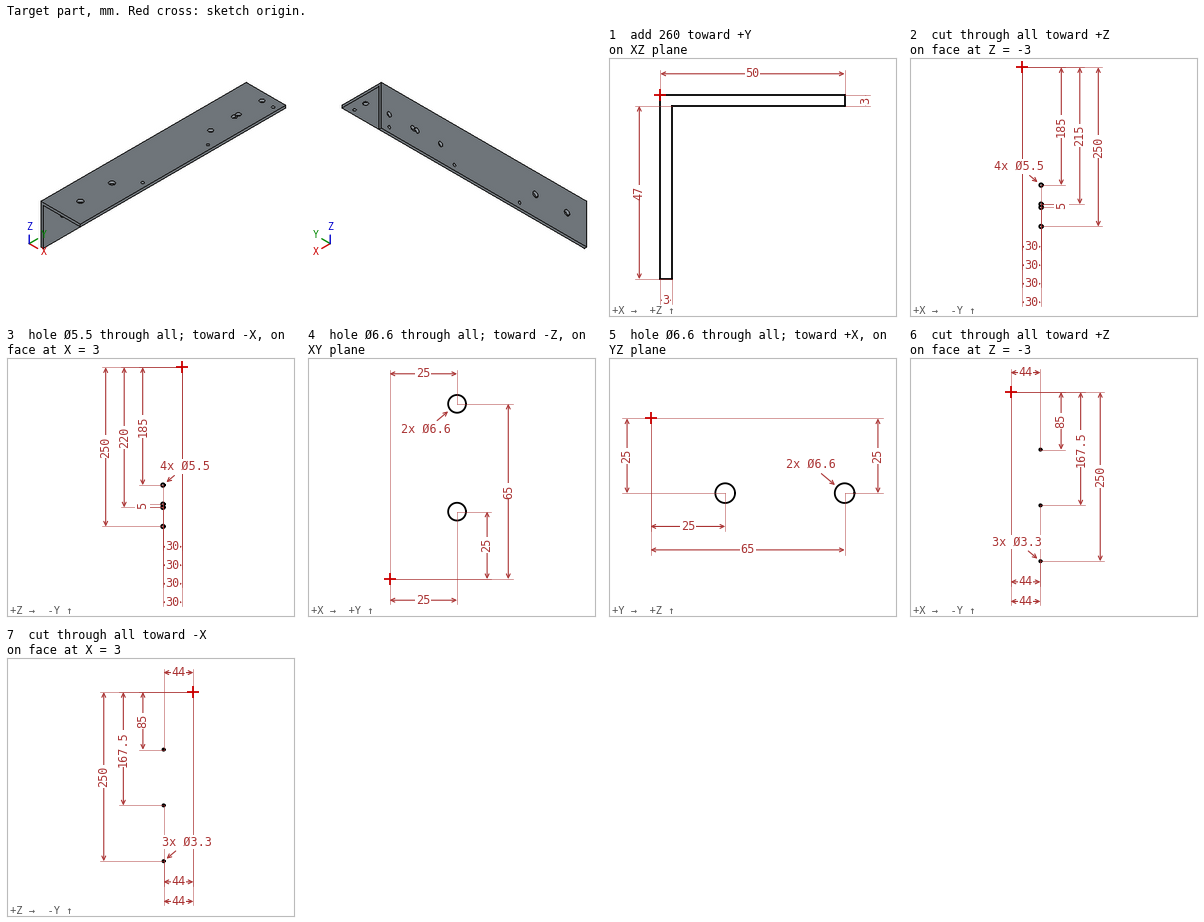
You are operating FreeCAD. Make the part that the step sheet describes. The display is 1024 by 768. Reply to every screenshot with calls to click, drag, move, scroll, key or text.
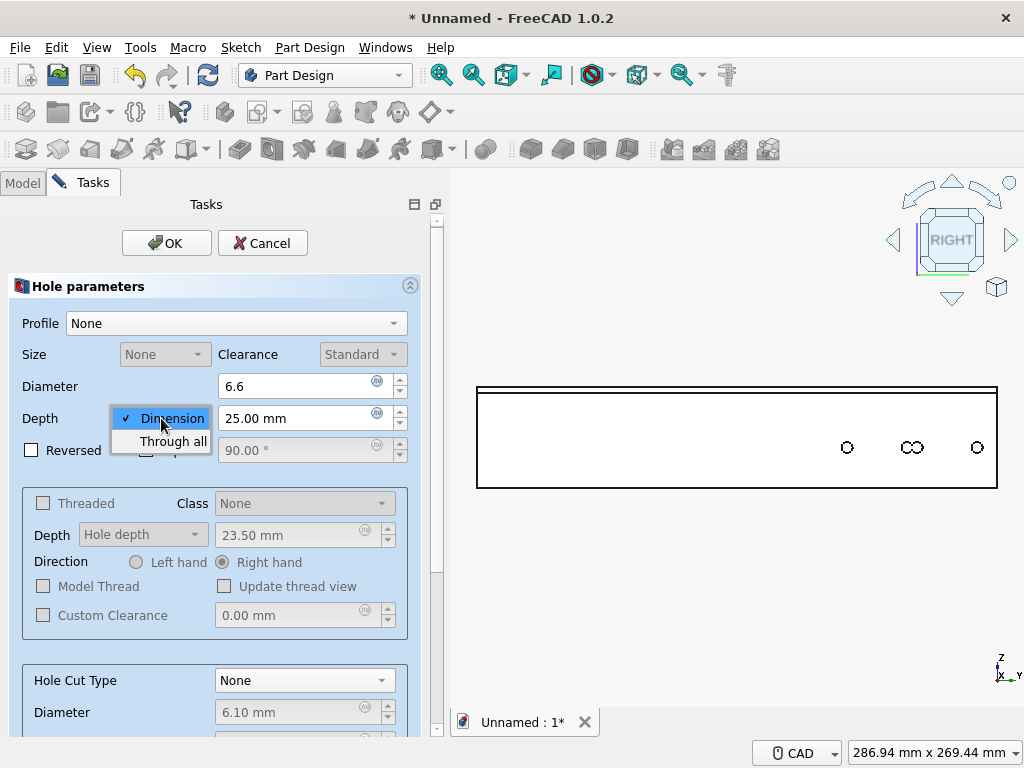
click(160, 442)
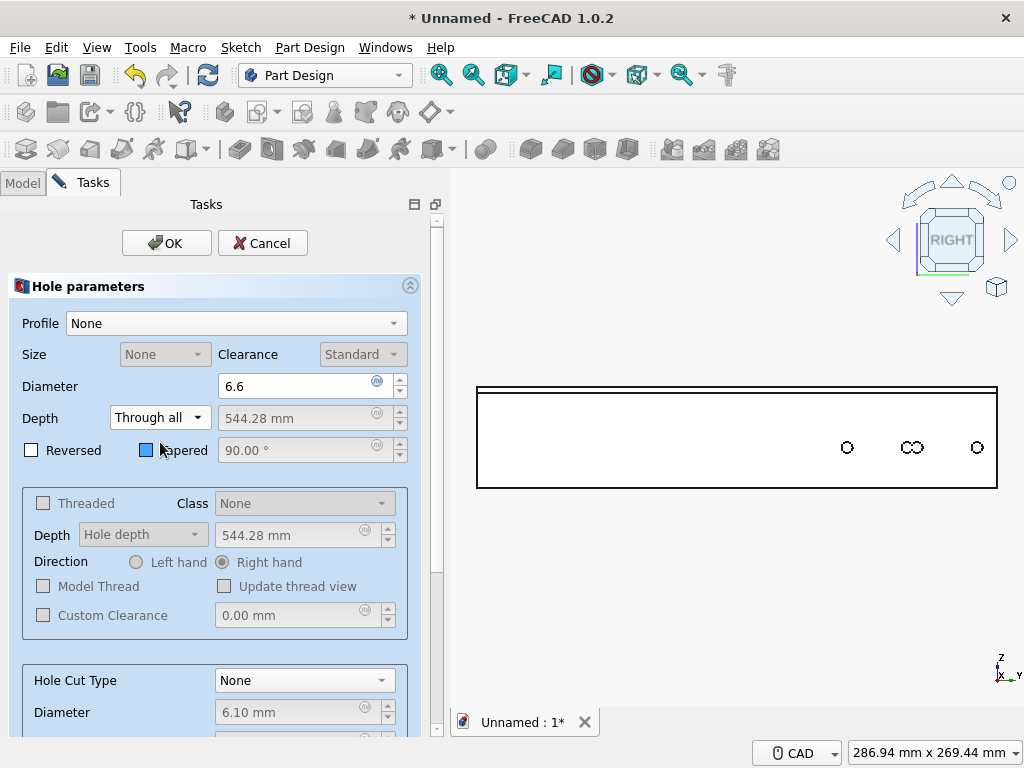
click(167, 243)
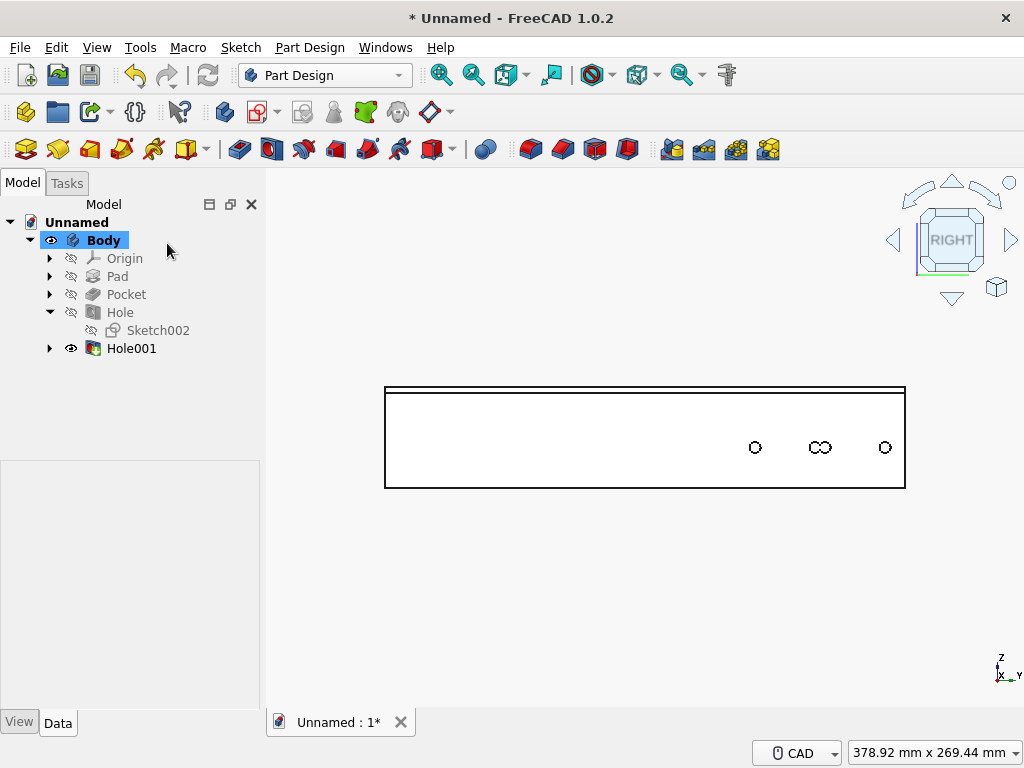
click(258, 112)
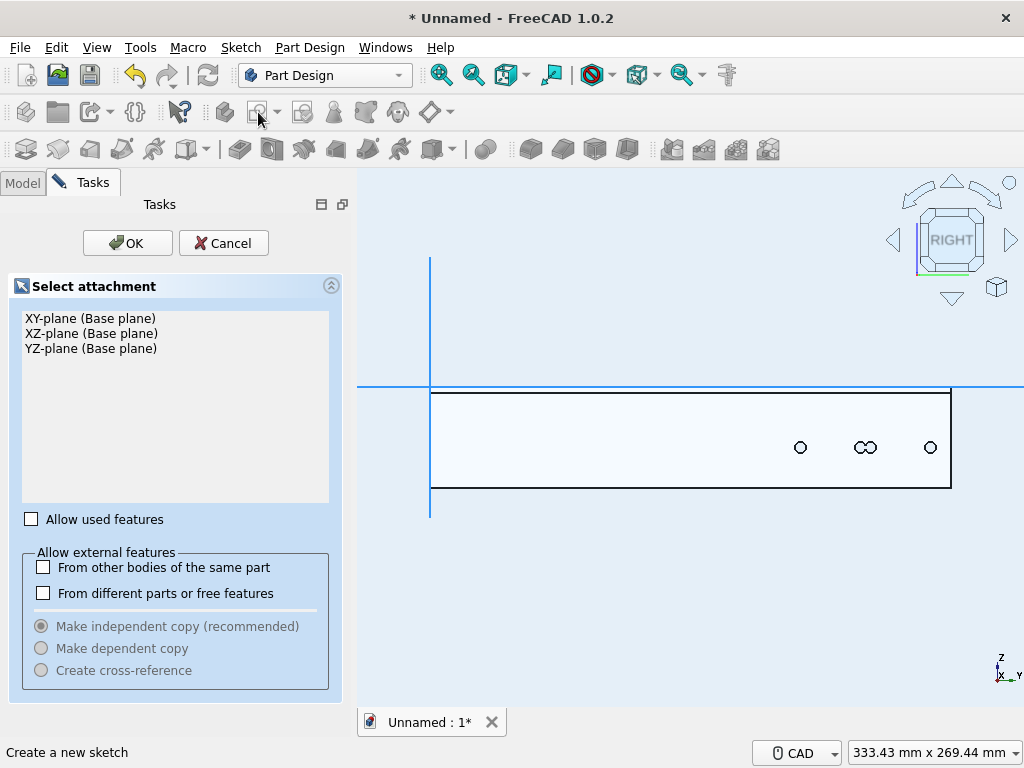
click(82, 348)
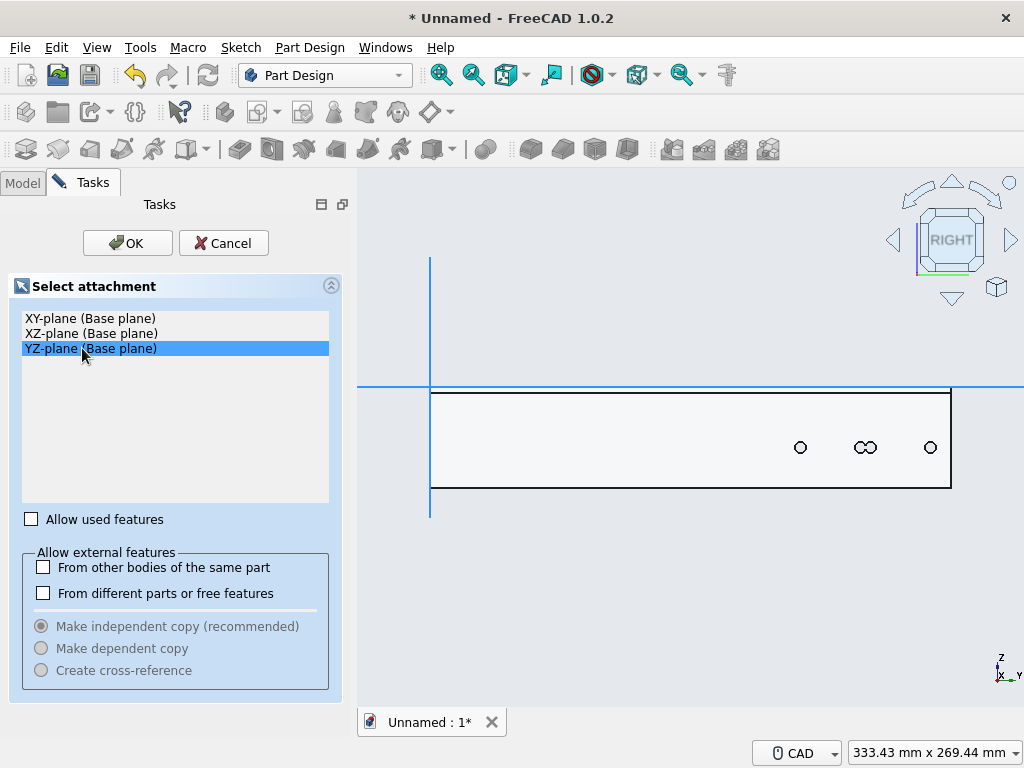
click(128, 243)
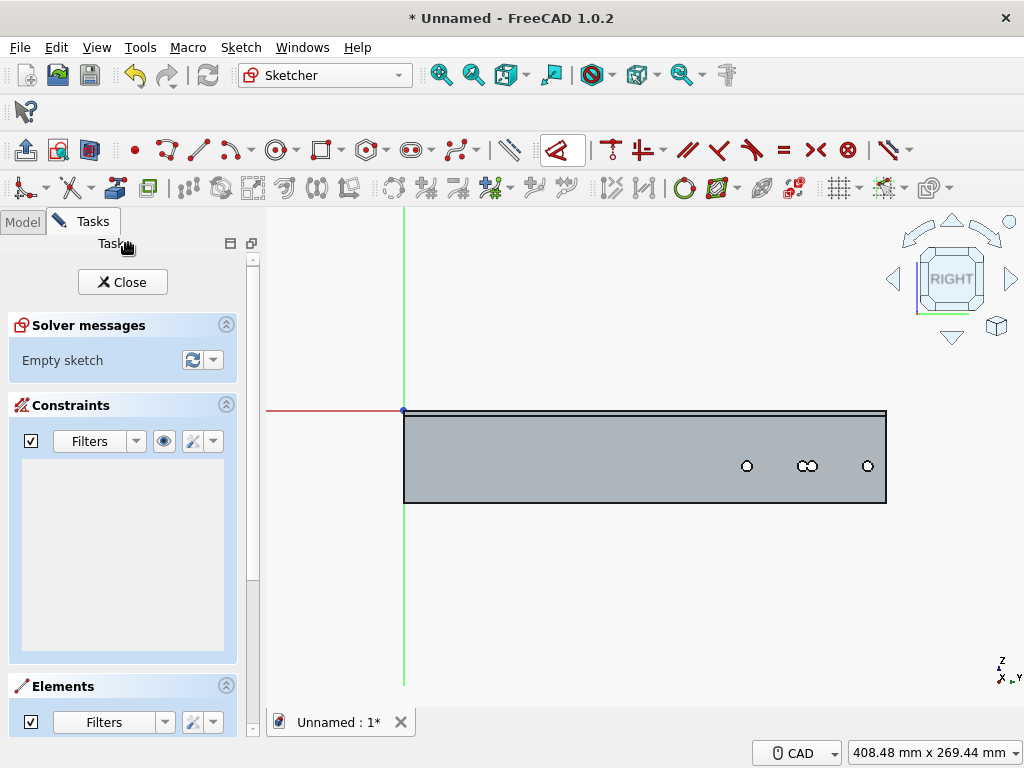
key(q)
key(s)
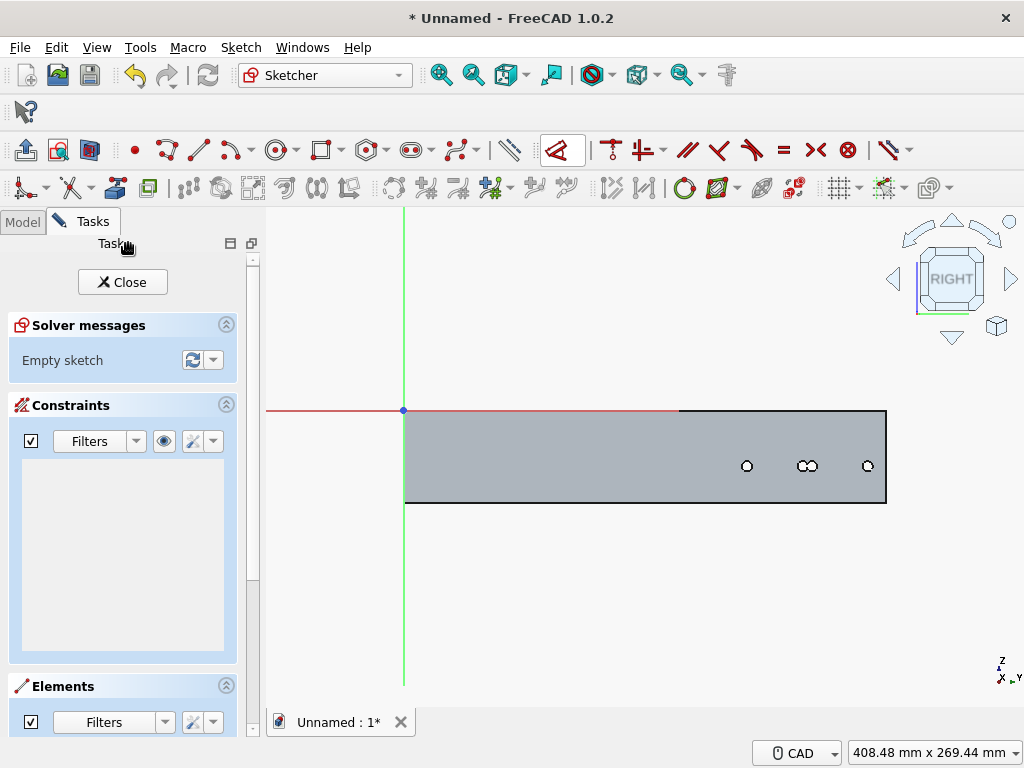
scroll(420, 428, up, 6)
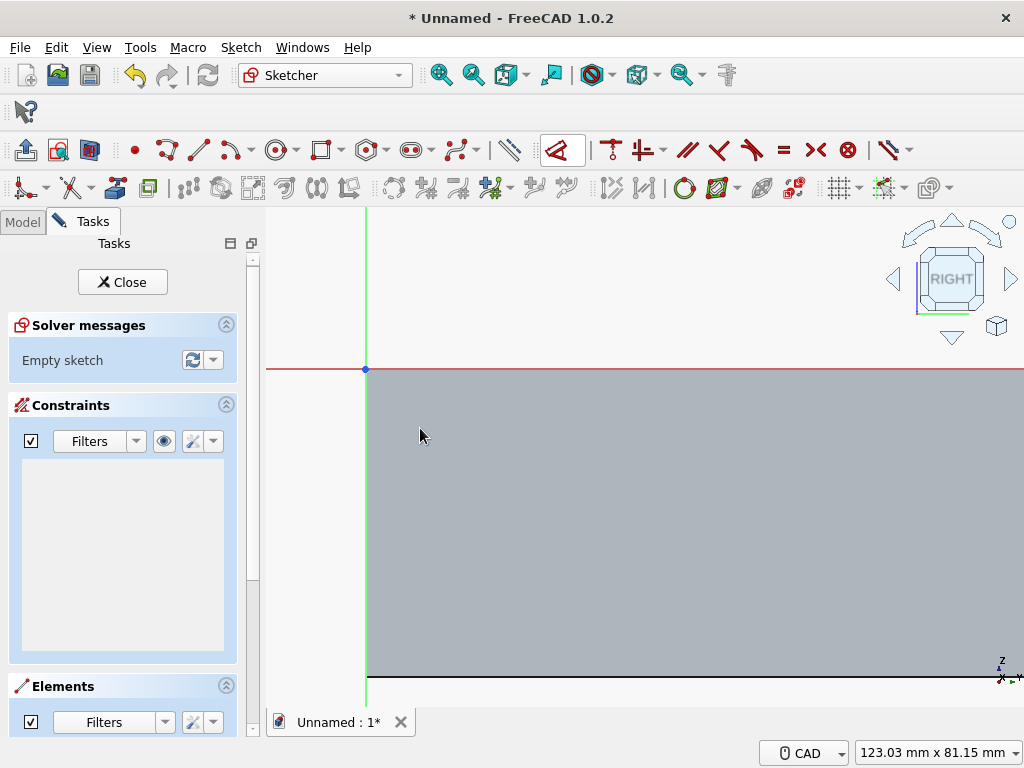
key(g)
key(c)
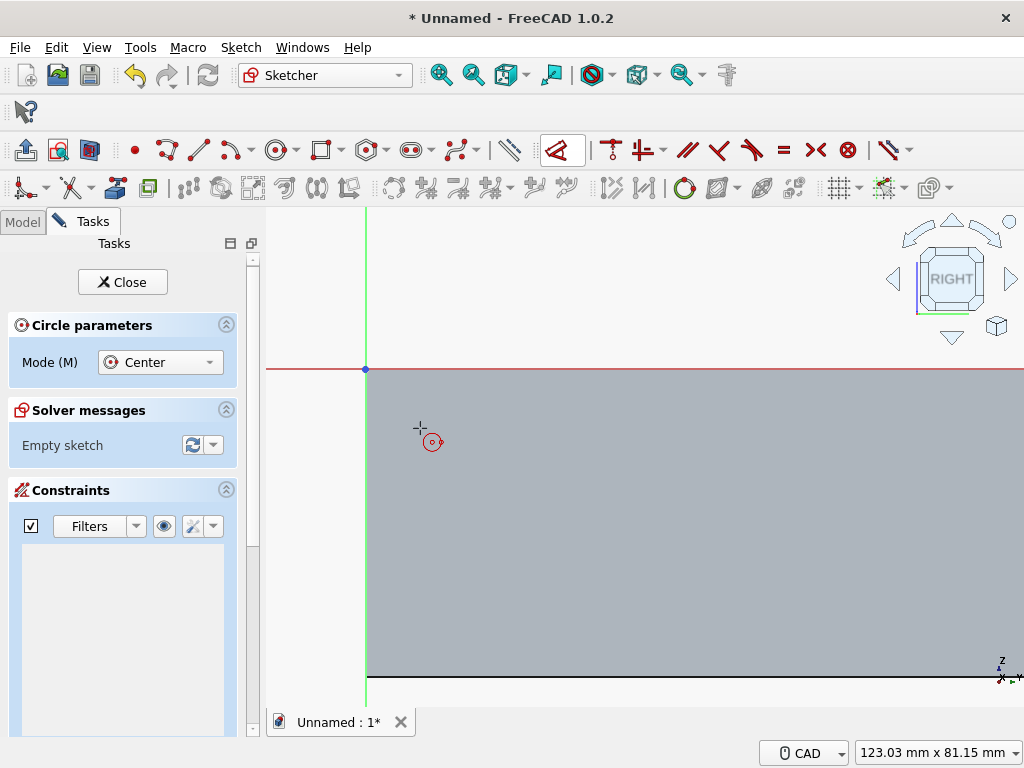
click(766, 523)
click(780, 509)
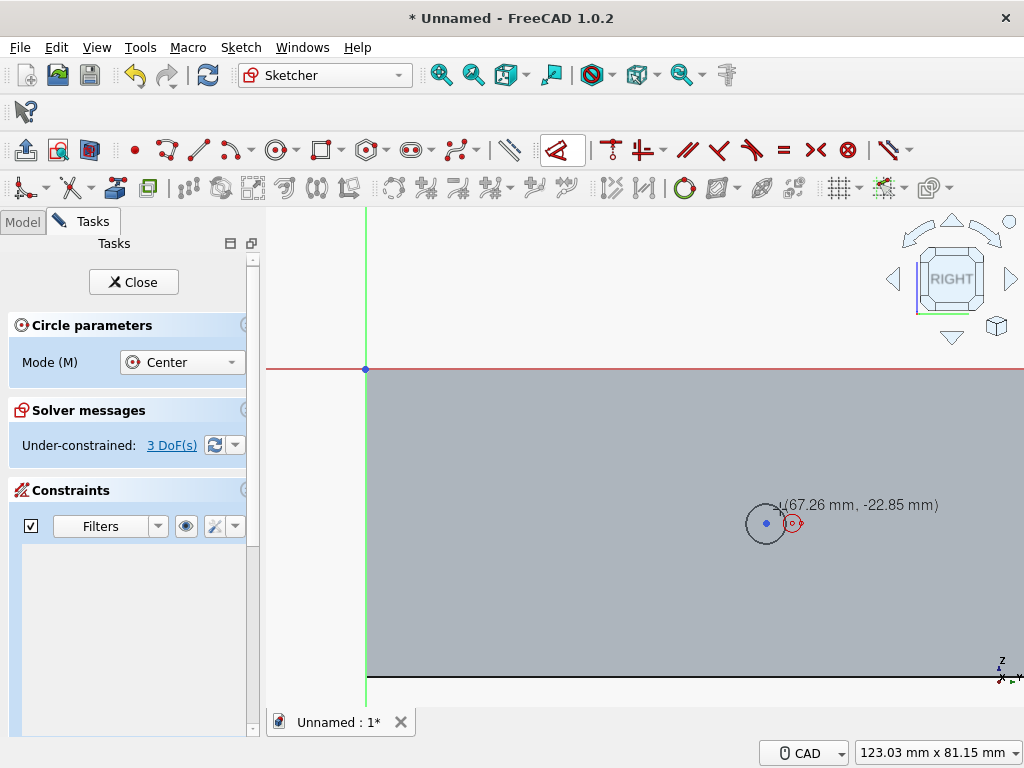
click(520, 523)
click(534, 509)
key(Escape)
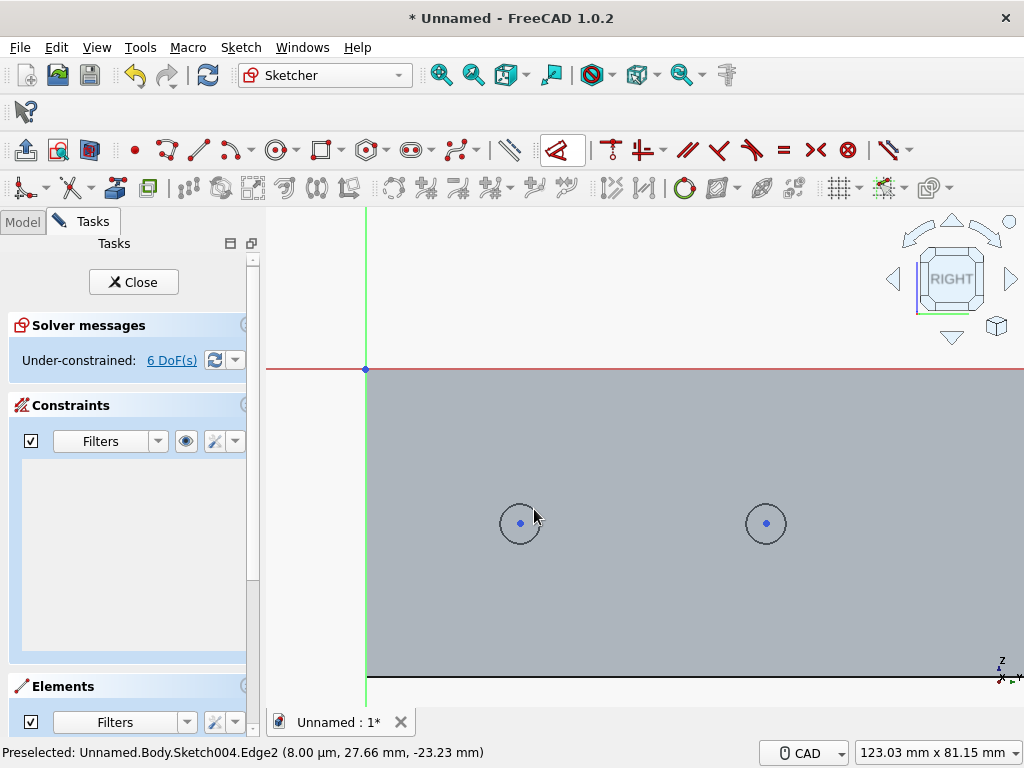
click(780, 510)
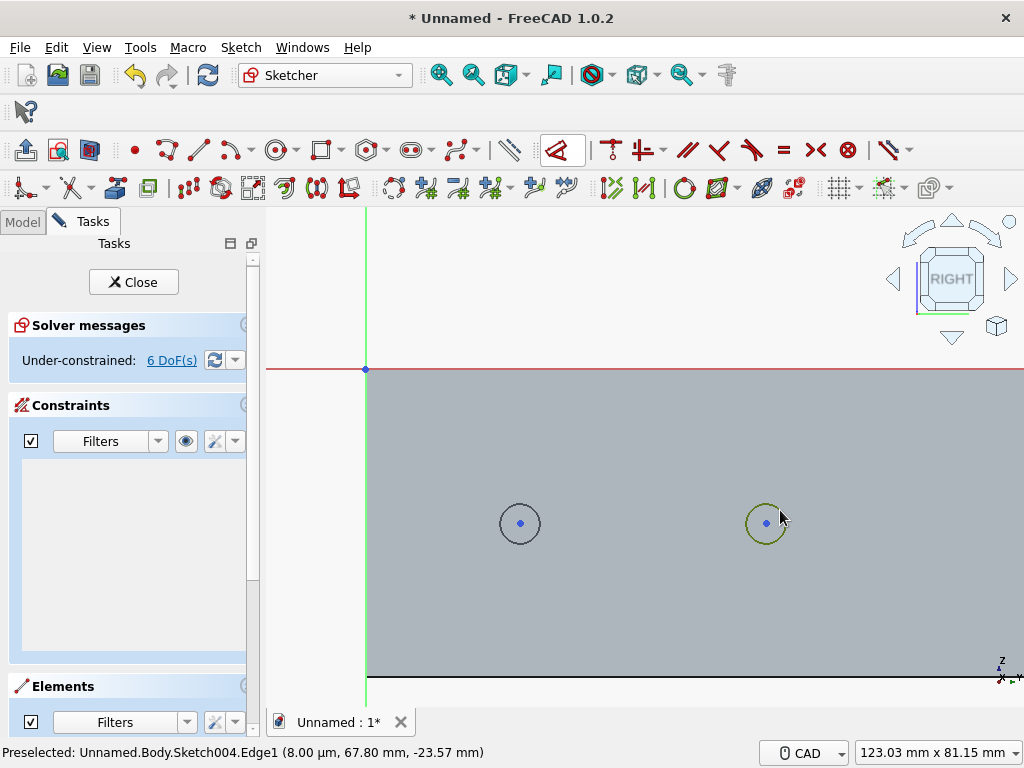
click(534, 510)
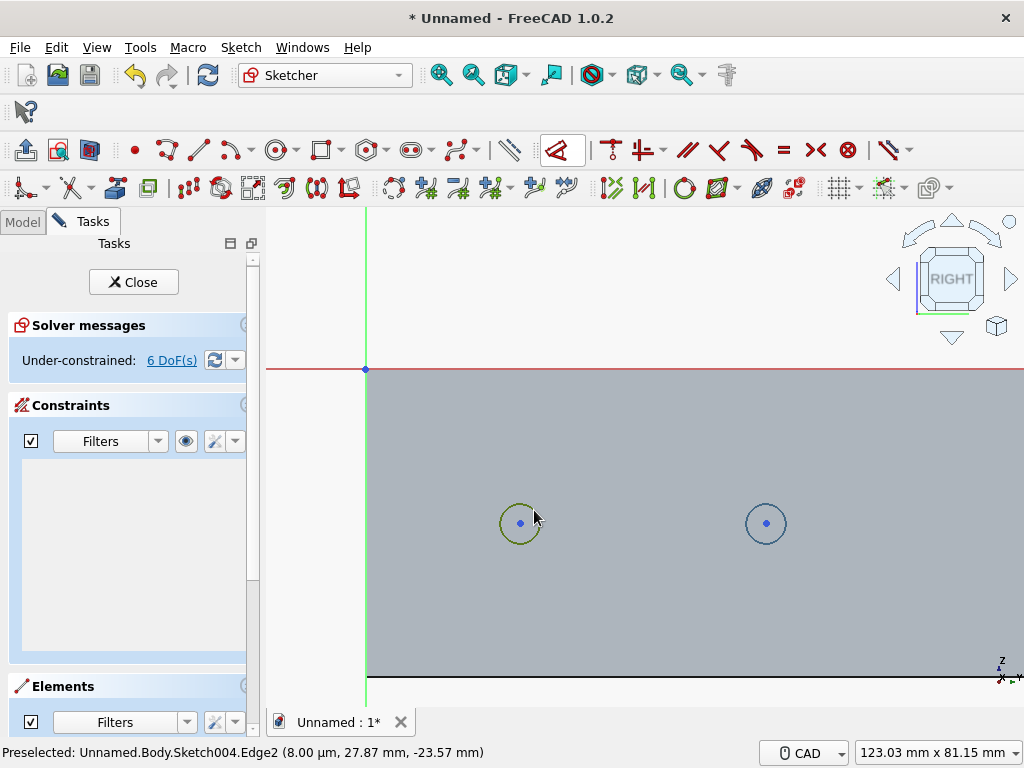
key(e)